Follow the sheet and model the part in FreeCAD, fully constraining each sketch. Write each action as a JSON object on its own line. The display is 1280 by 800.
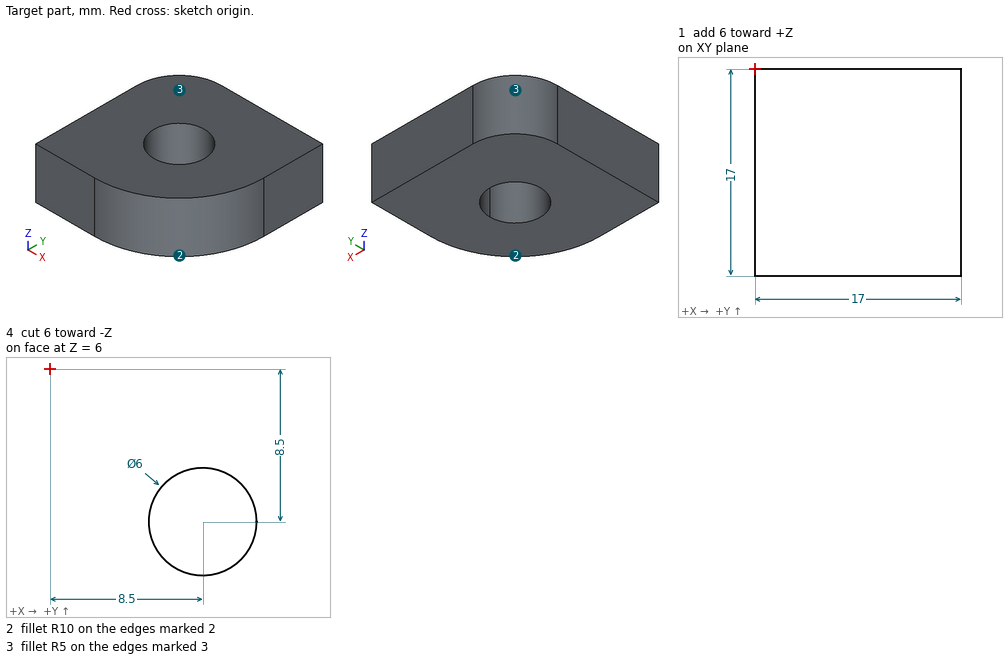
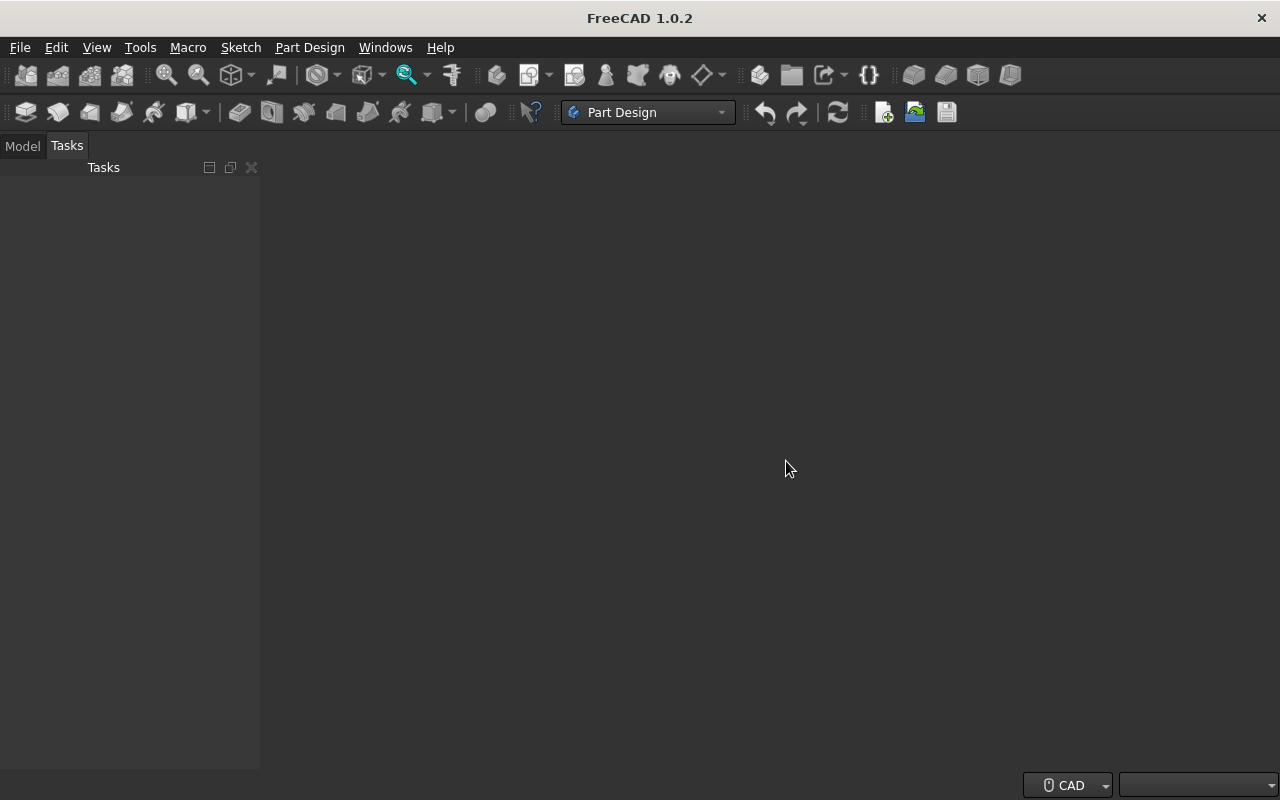
{"action": "left_click", "coordinate": [884, 112]}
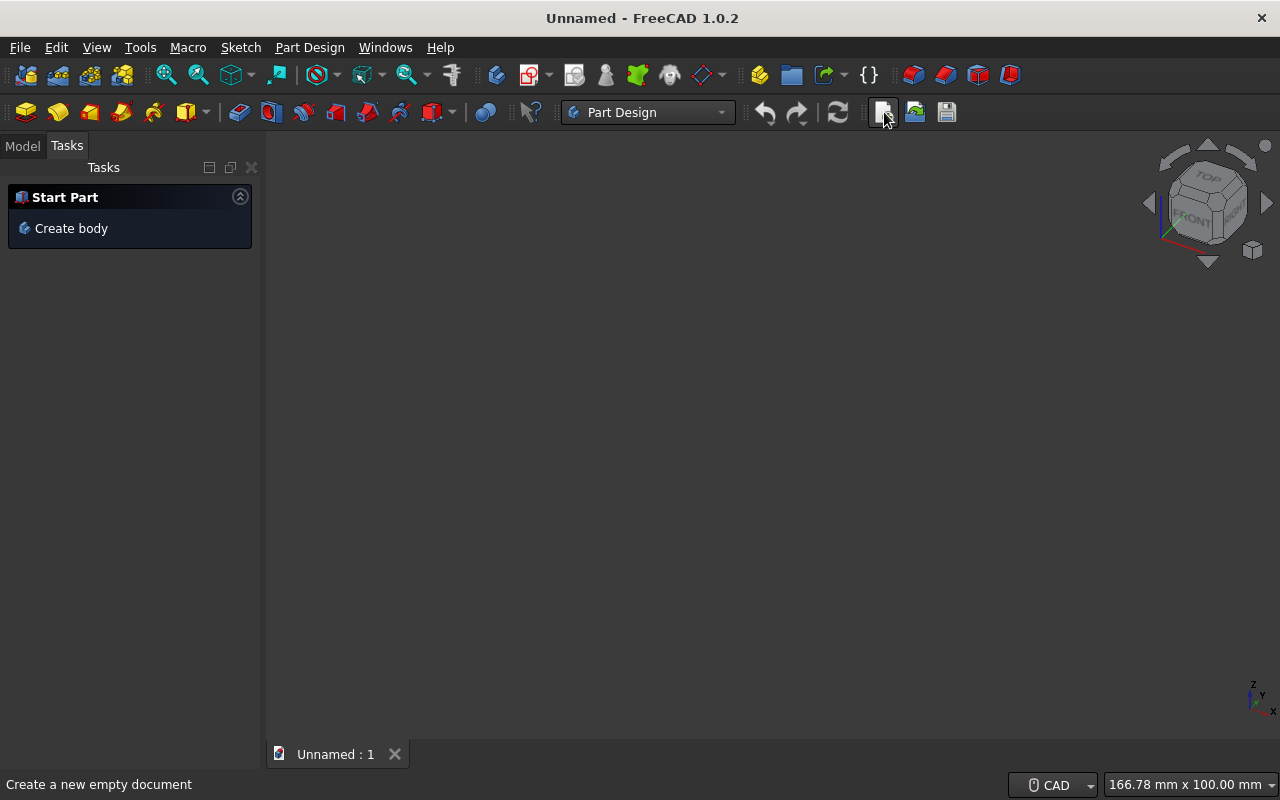
{"action": "left_click", "coordinate": [530, 76]}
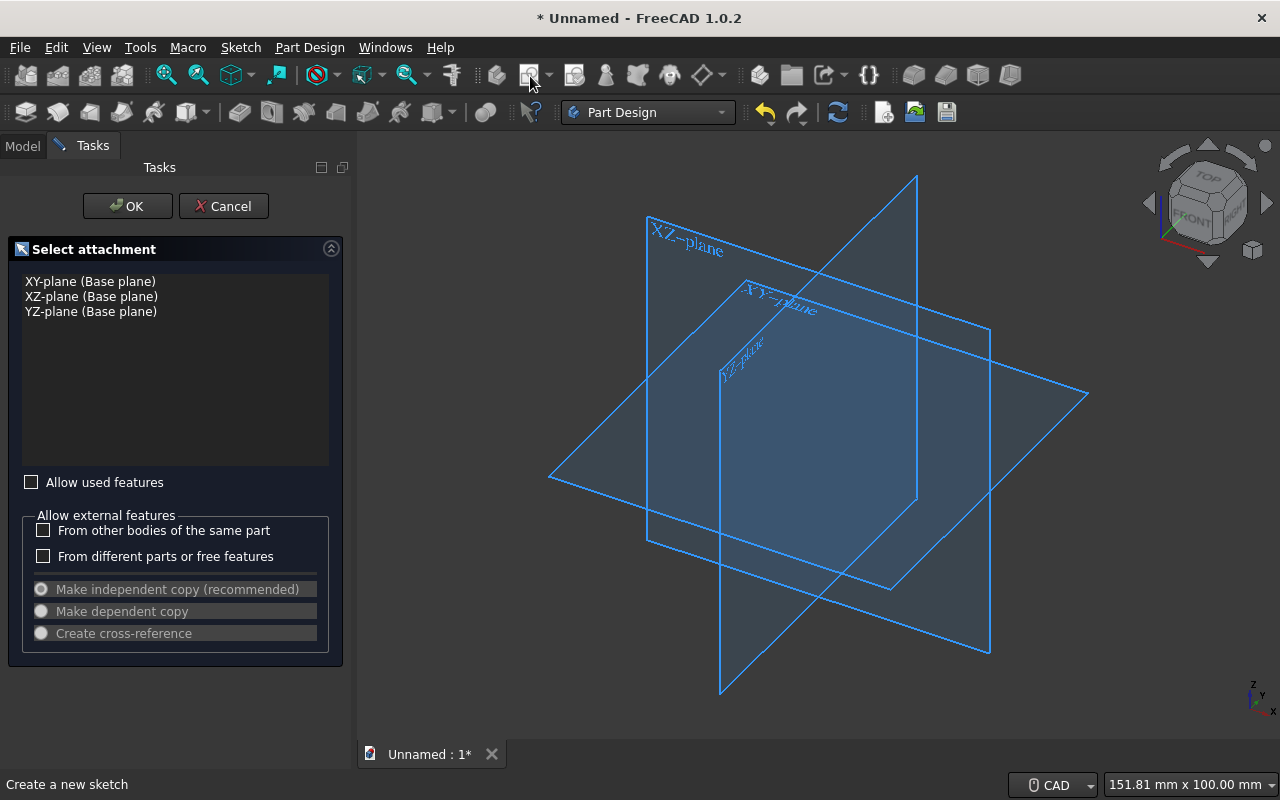
{"action": "left_click", "coordinate": [82, 282]}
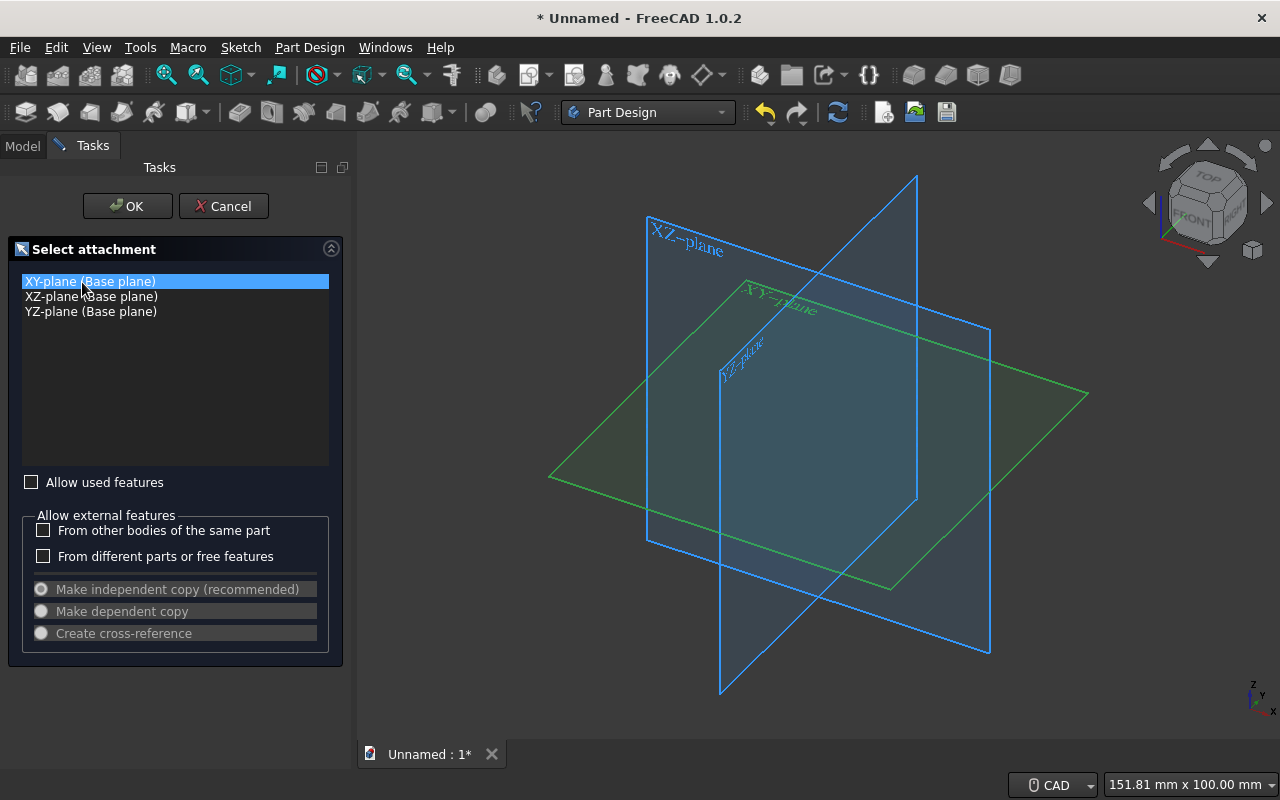
{"action": "left_click", "coordinate": [128, 206]}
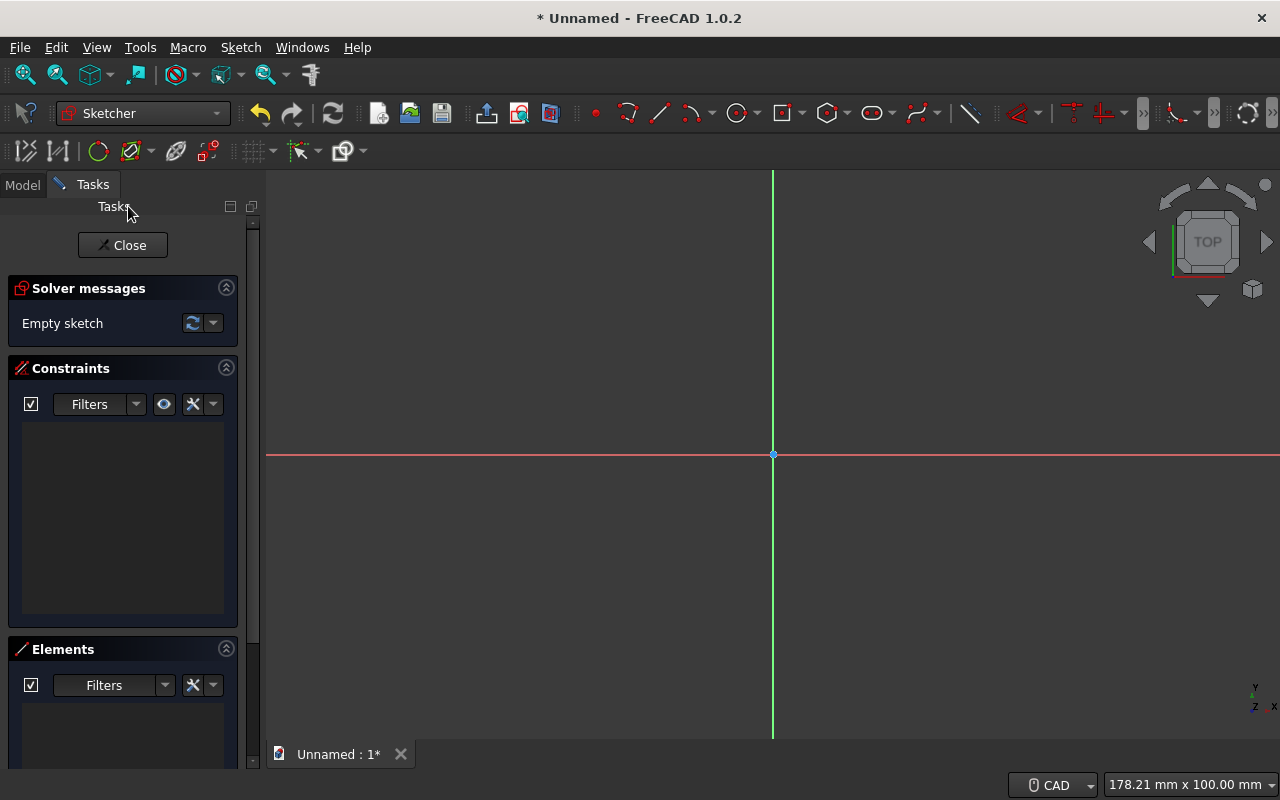
{"action": "scroll", "coordinate": [860, 519], "scroll_direction": "up", "scroll_amount": 7}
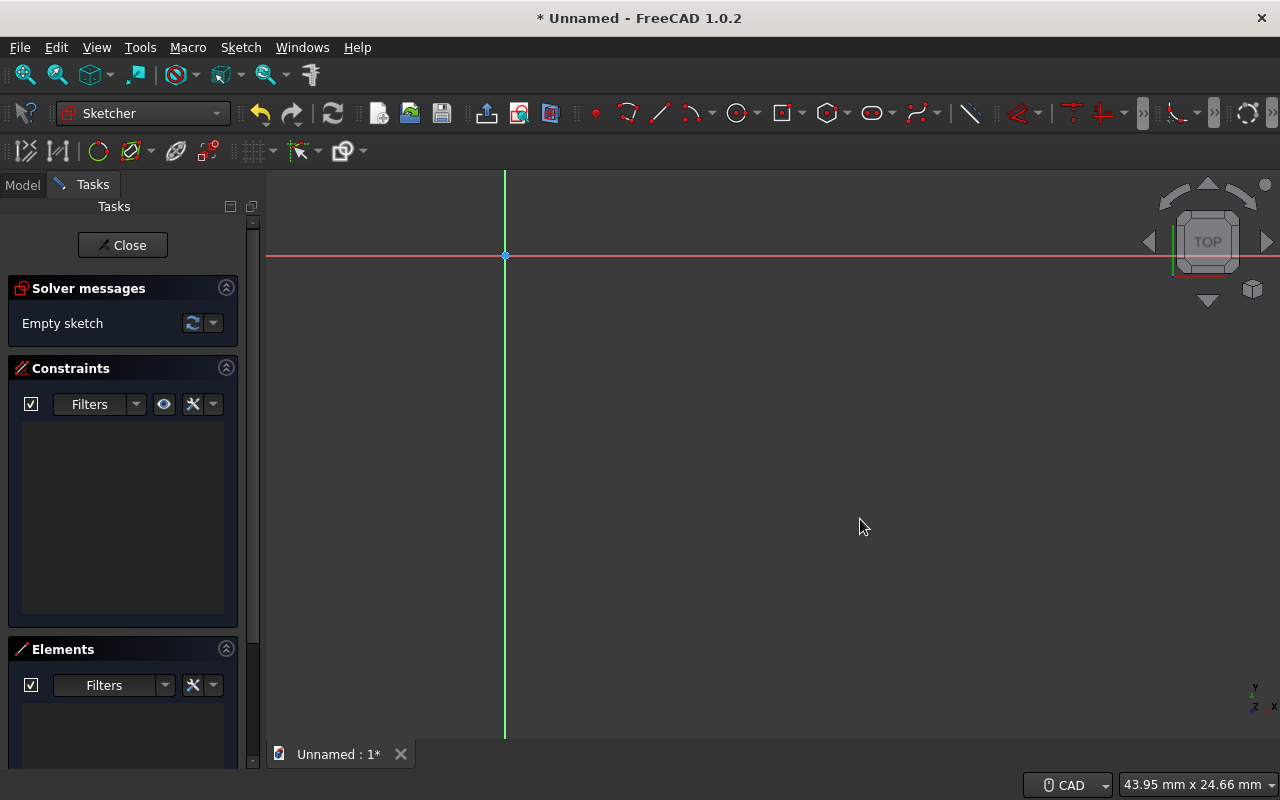
{"action": "key", "text": "g r"}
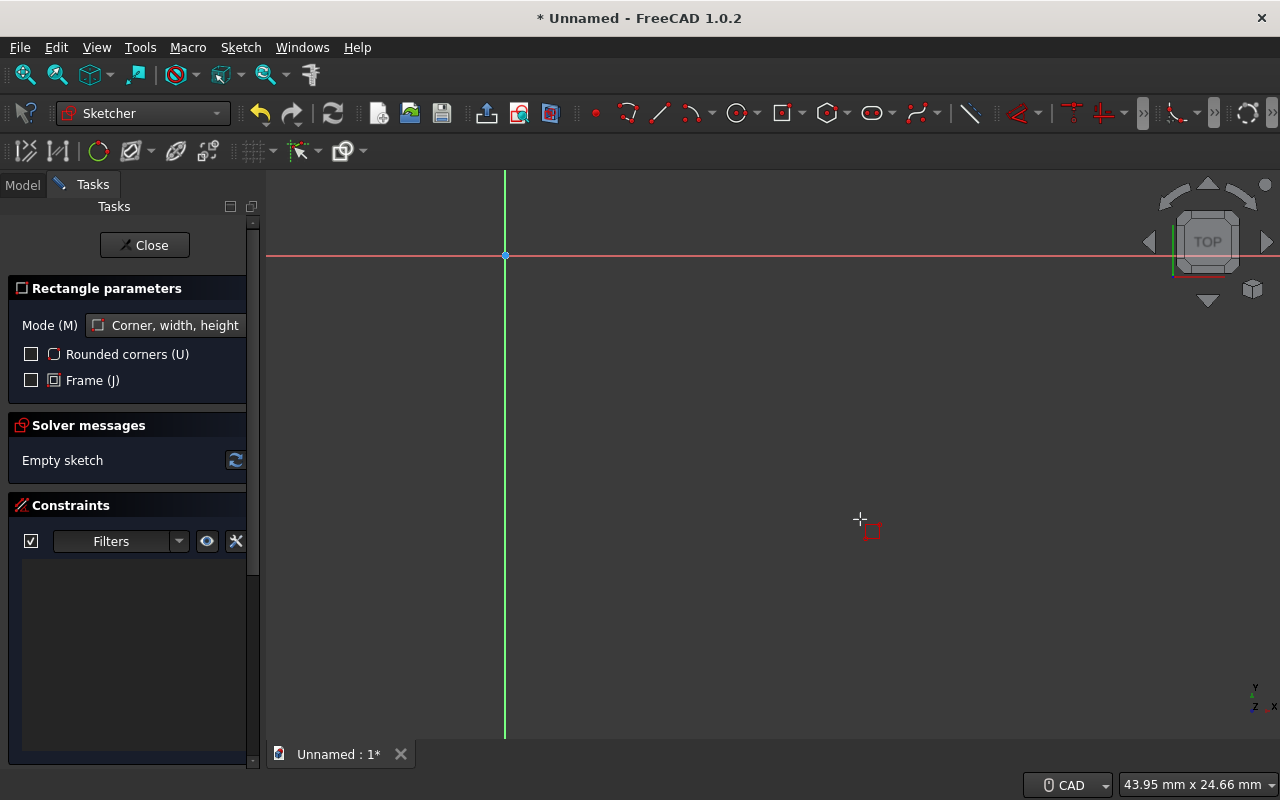
{"action": "left_click", "coordinate": [505, 256]}
{"action": "left_click", "coordinate": [898, 648]}
{"action": "key", "text": "Escape"}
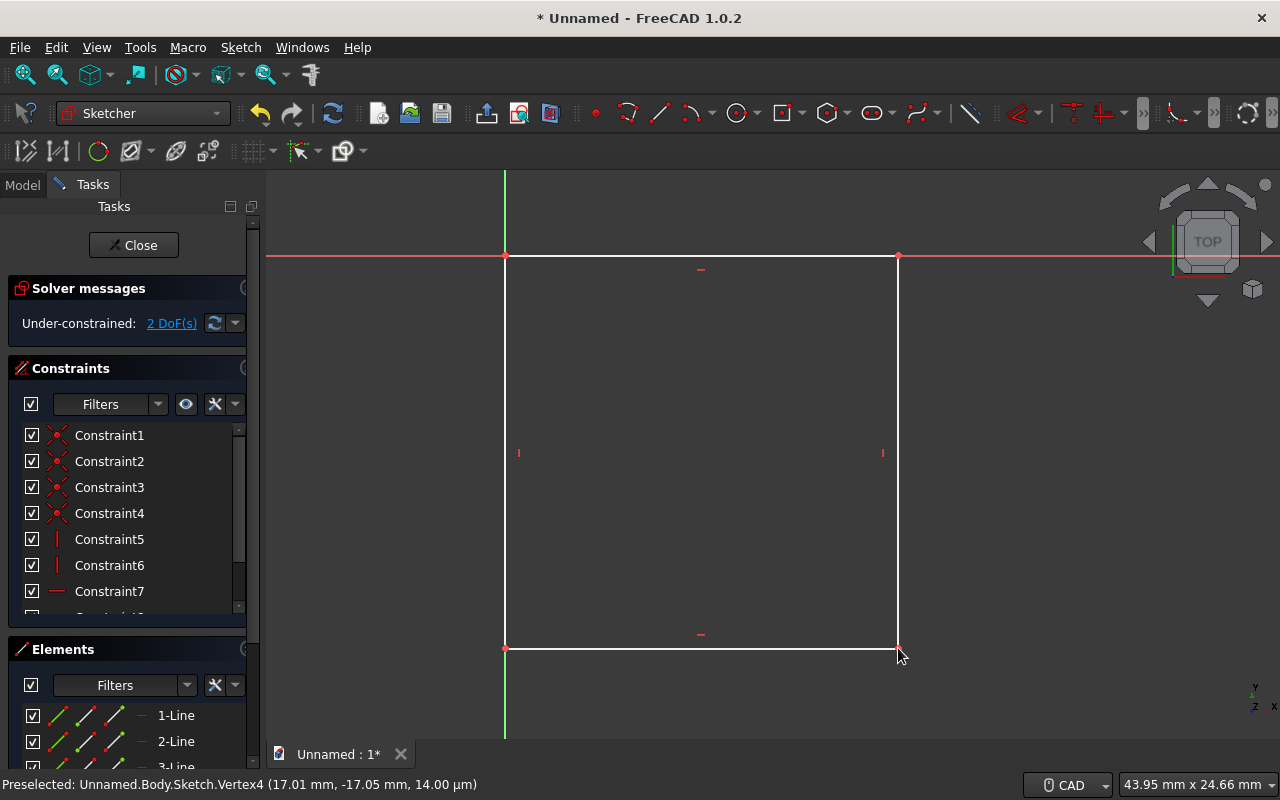
{"action": "left_click", "coordinate": [505, 374]}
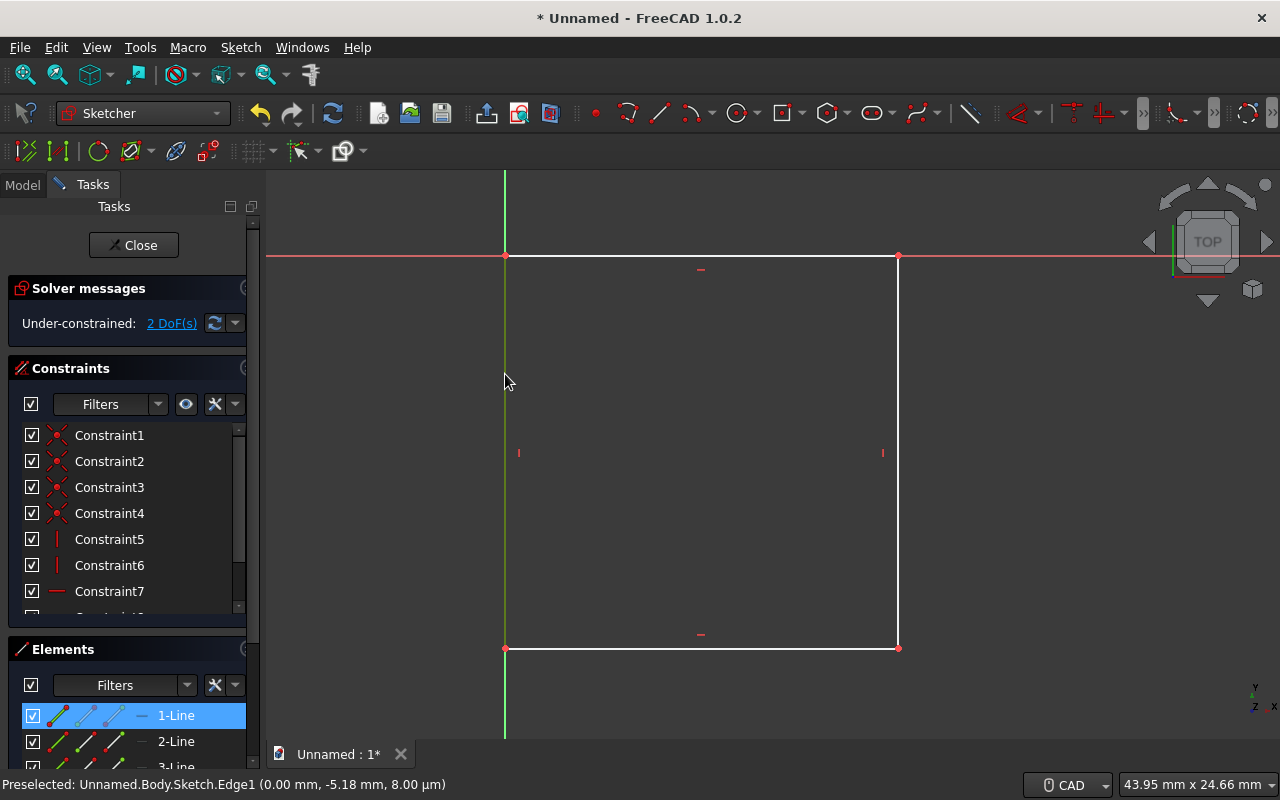
{"action": "key", "text": "i"}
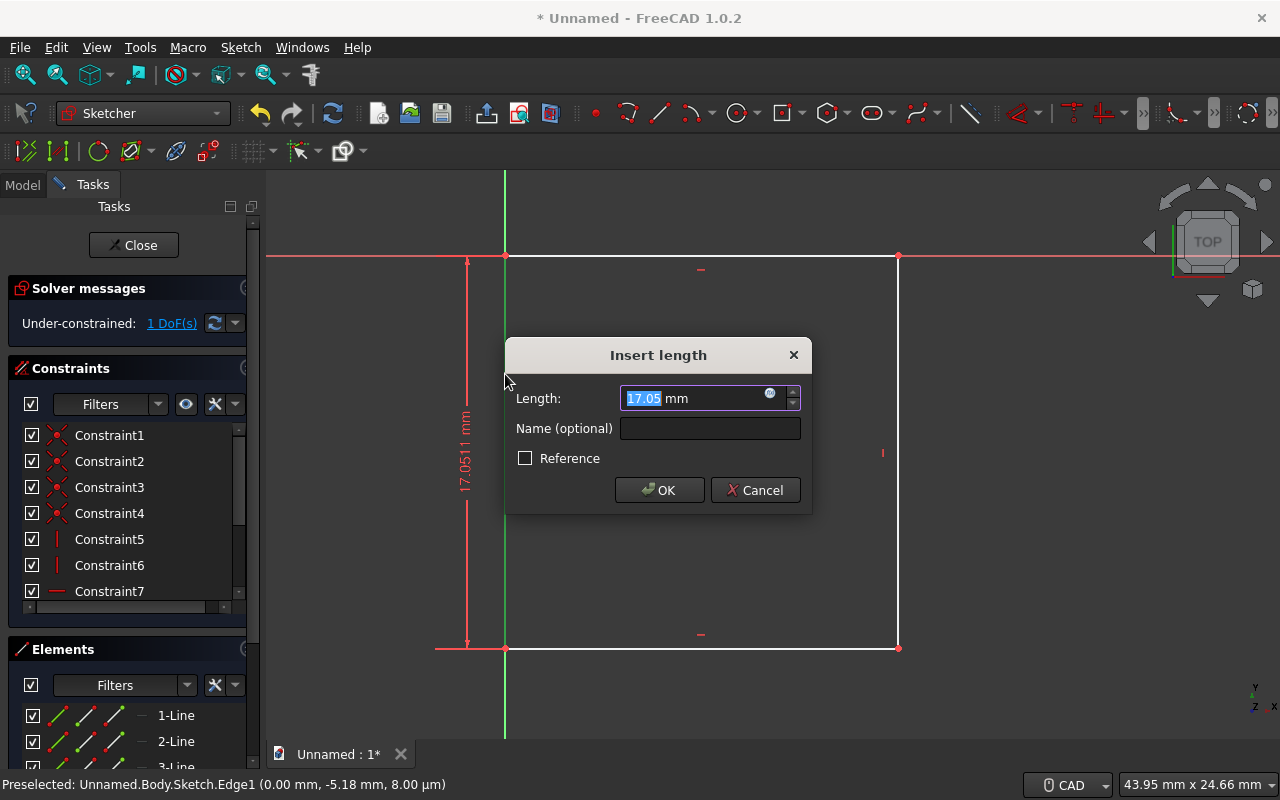
{"action": "type", "text": "17"}
{"action": "key", "text": "Return"}